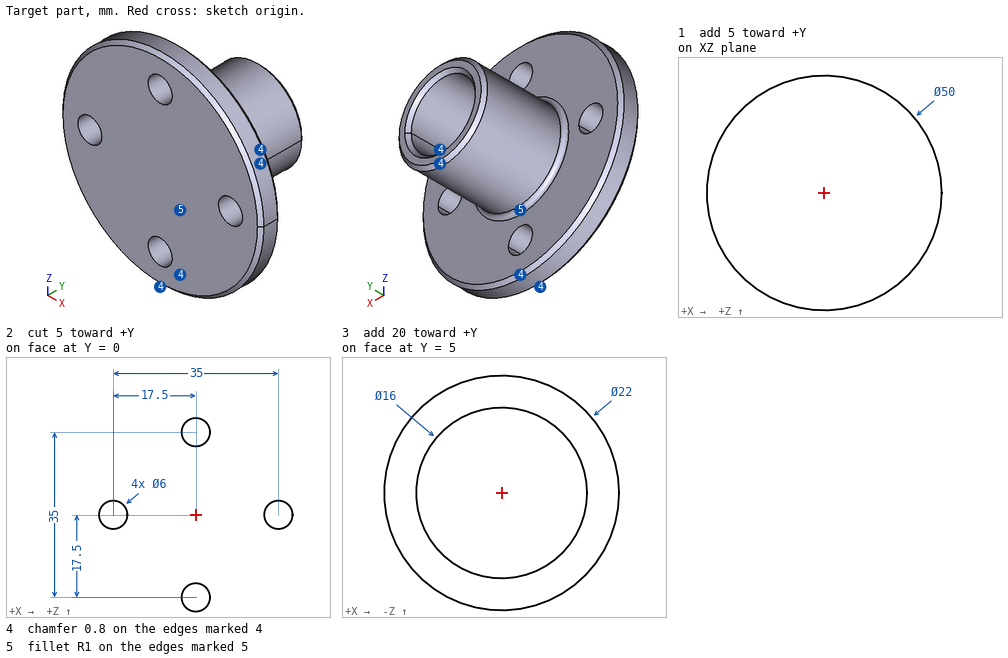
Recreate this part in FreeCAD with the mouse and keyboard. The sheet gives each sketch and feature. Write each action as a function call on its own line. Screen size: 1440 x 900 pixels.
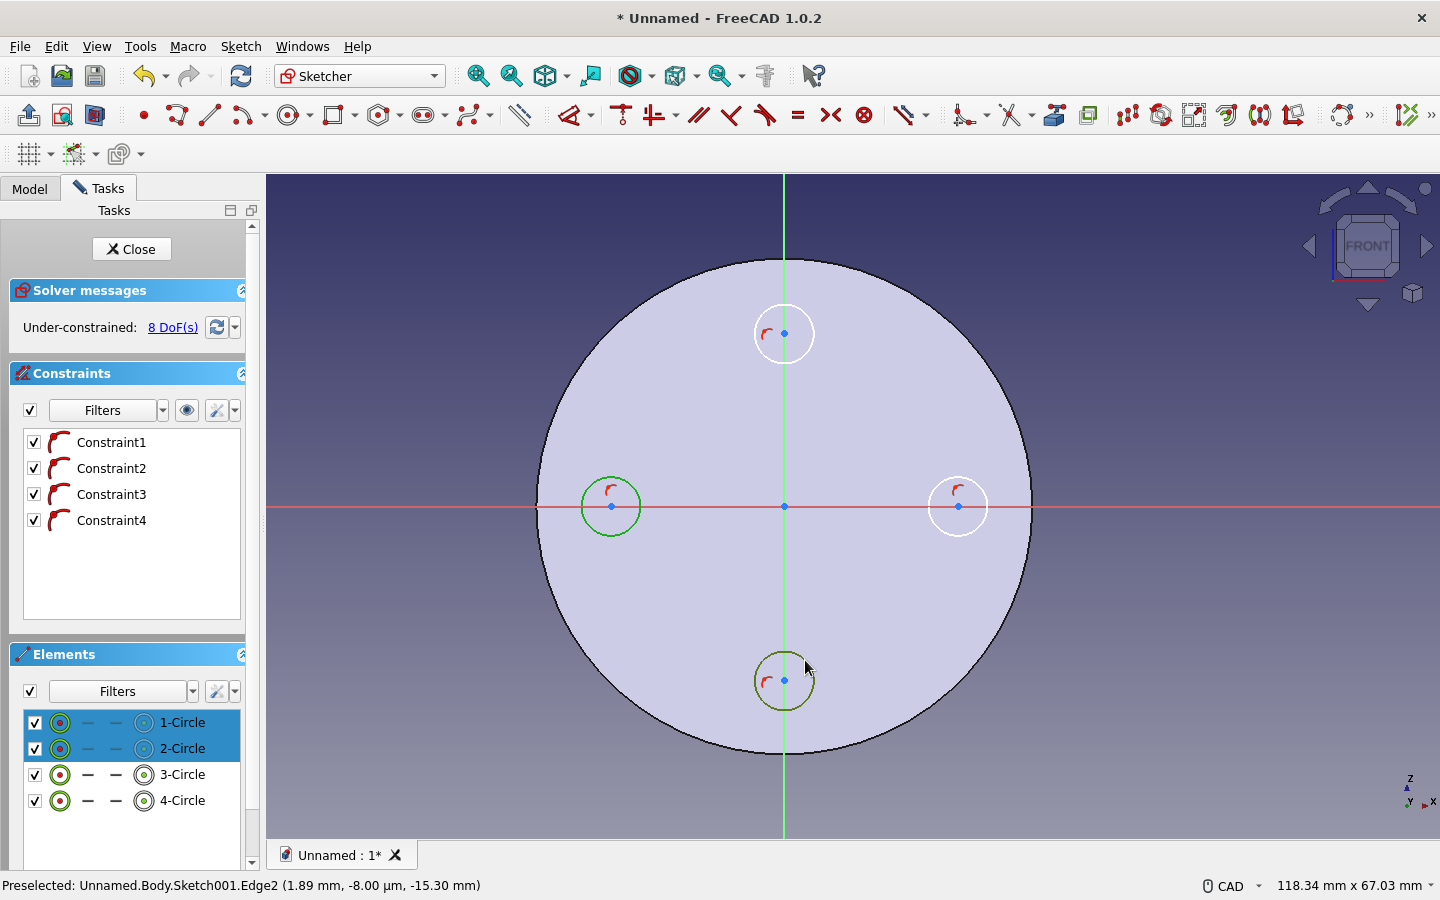
click(979, 486)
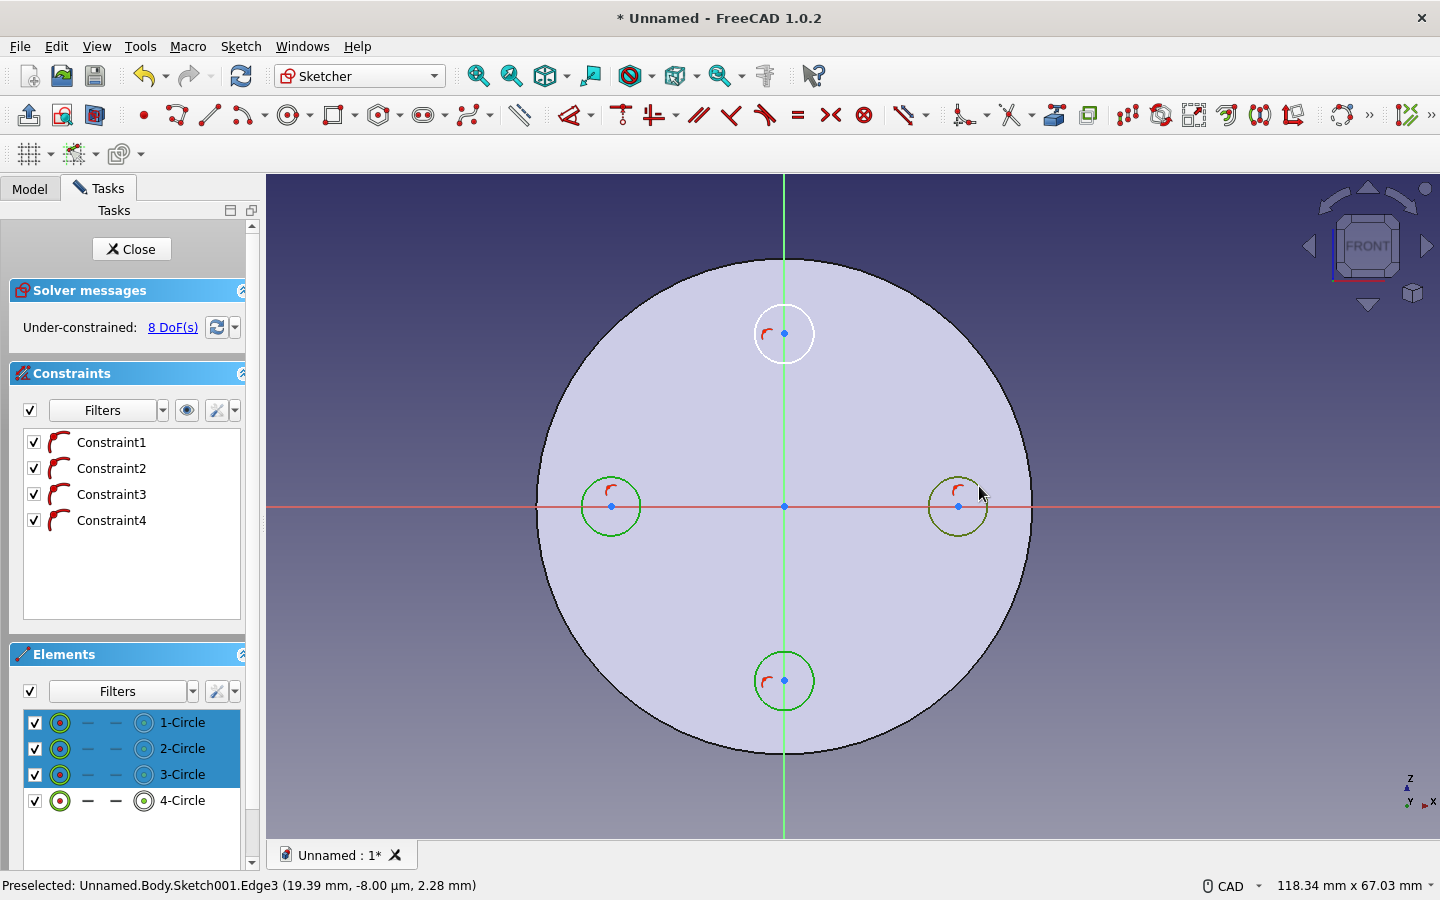
click(805, 313)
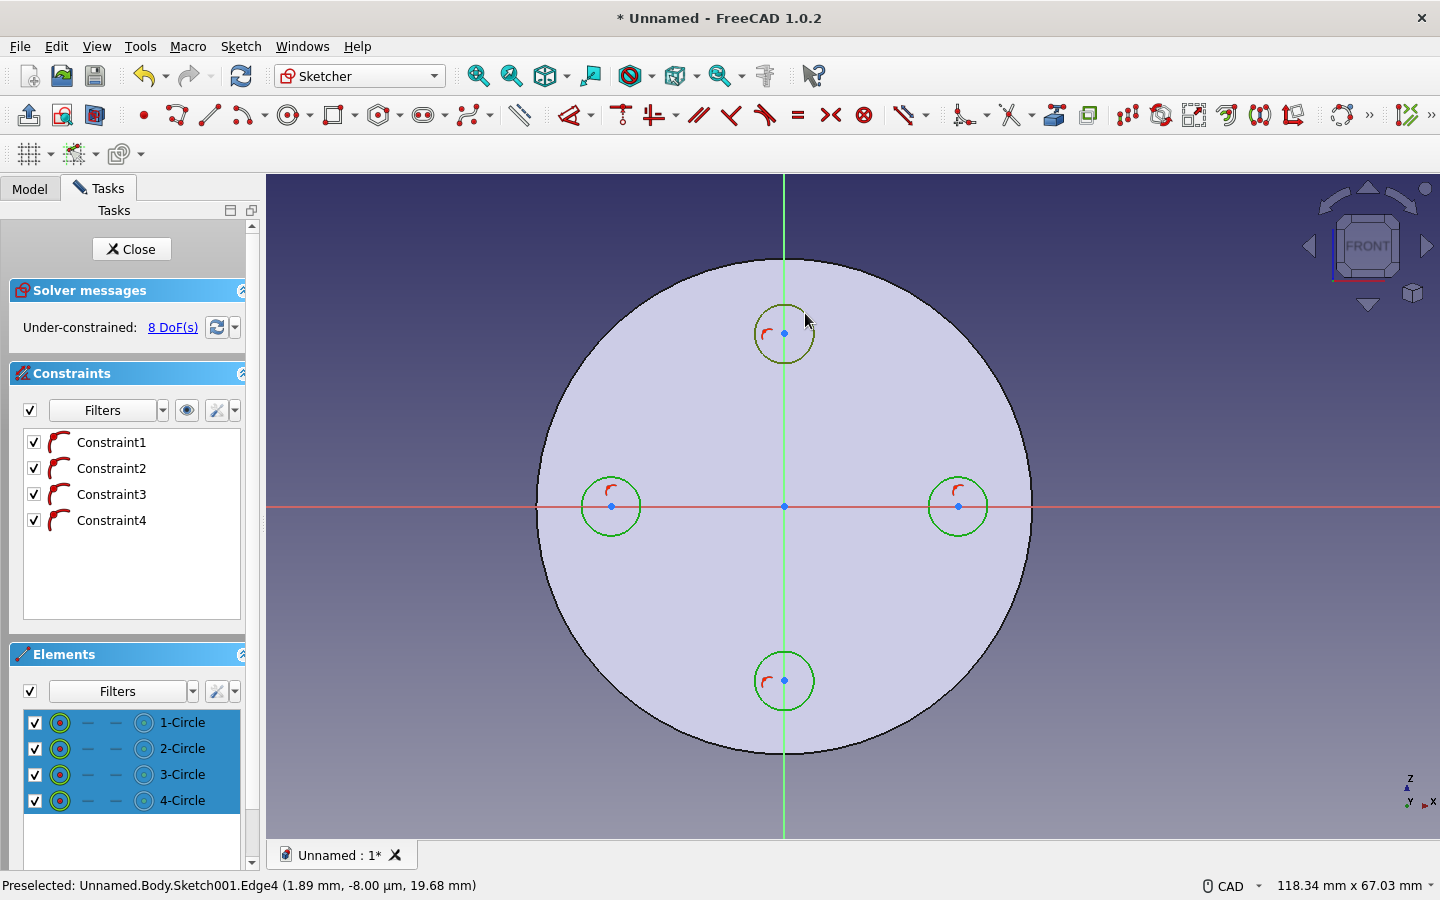
click(798, 116)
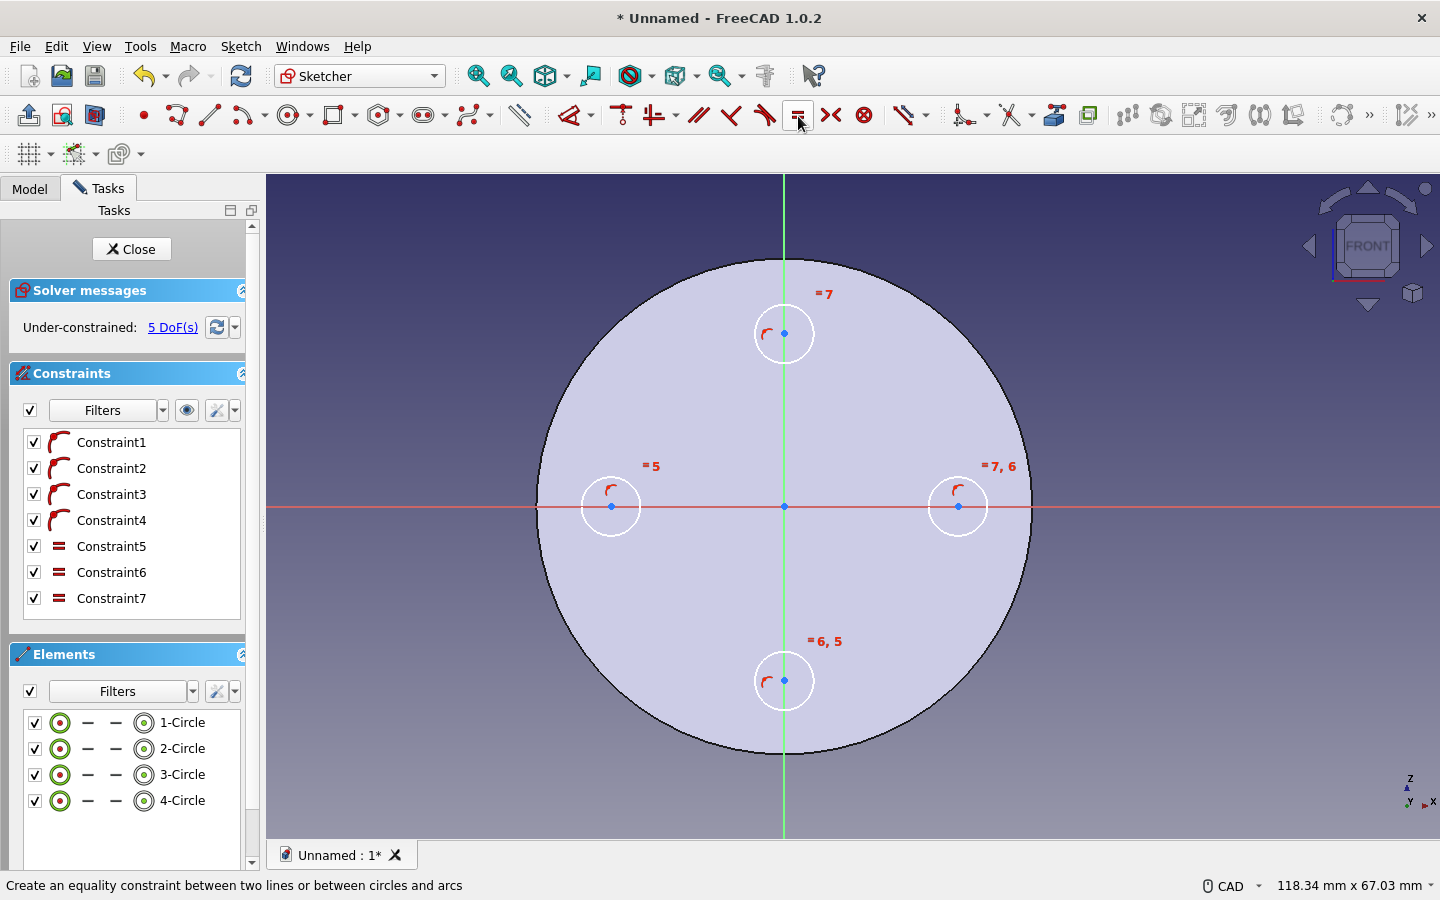
click(568, 116)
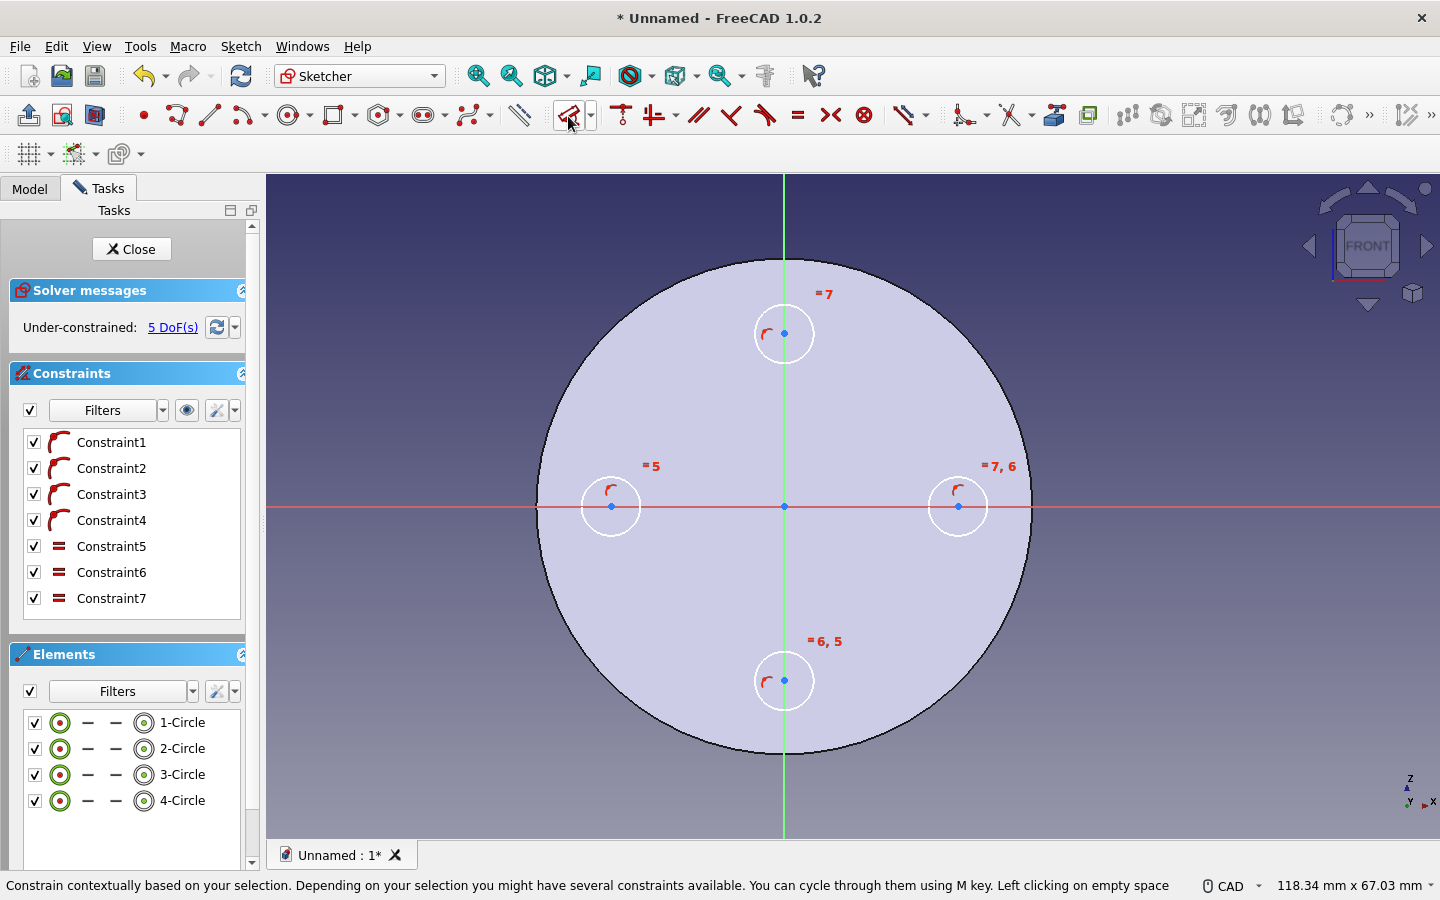
click(632, 486)
click(655, 464)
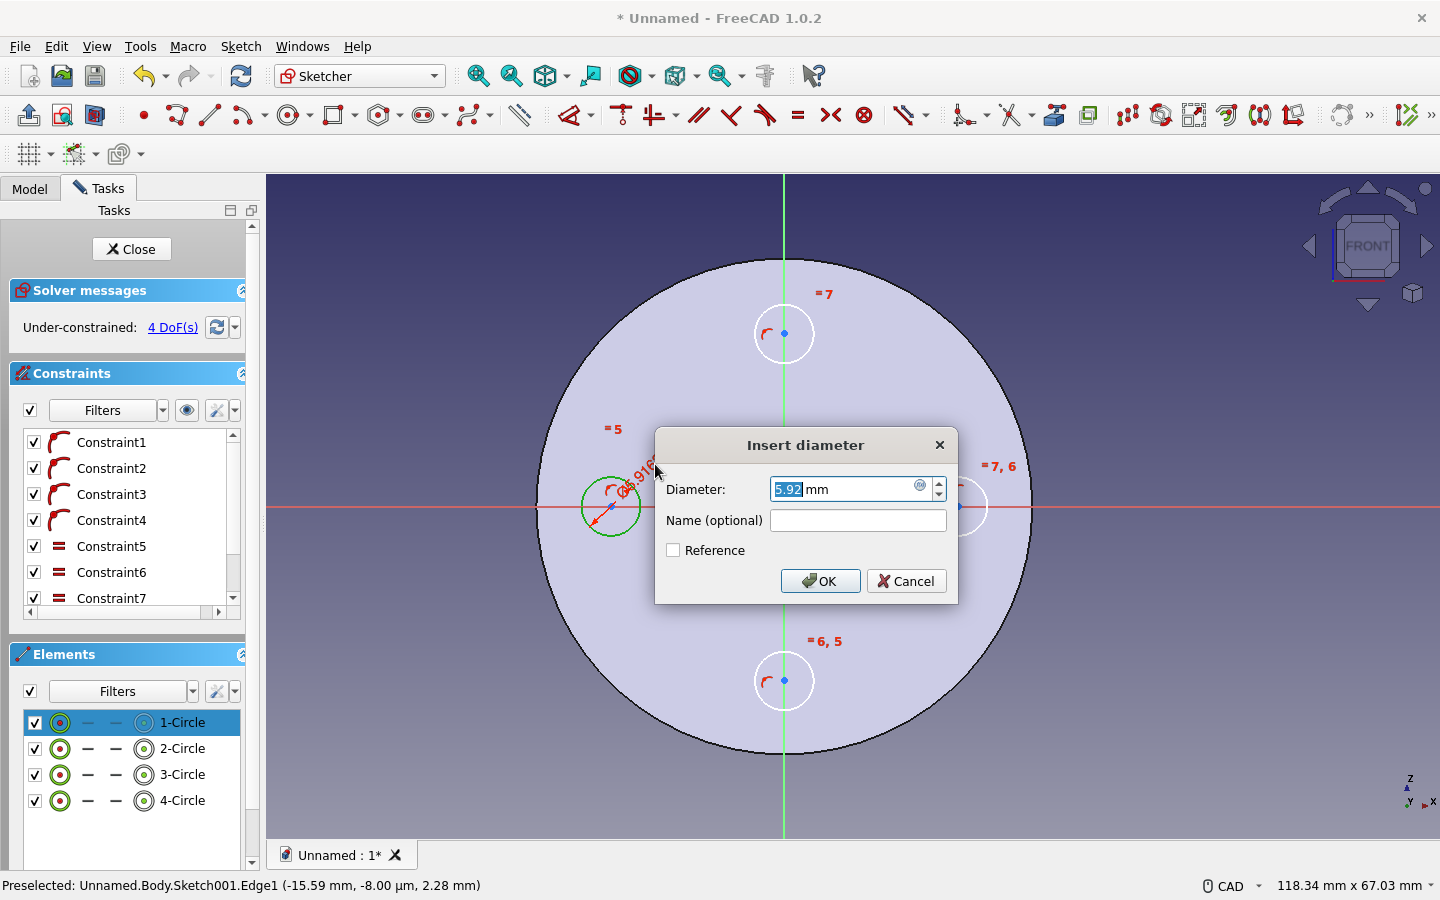
text(6)
key(Return)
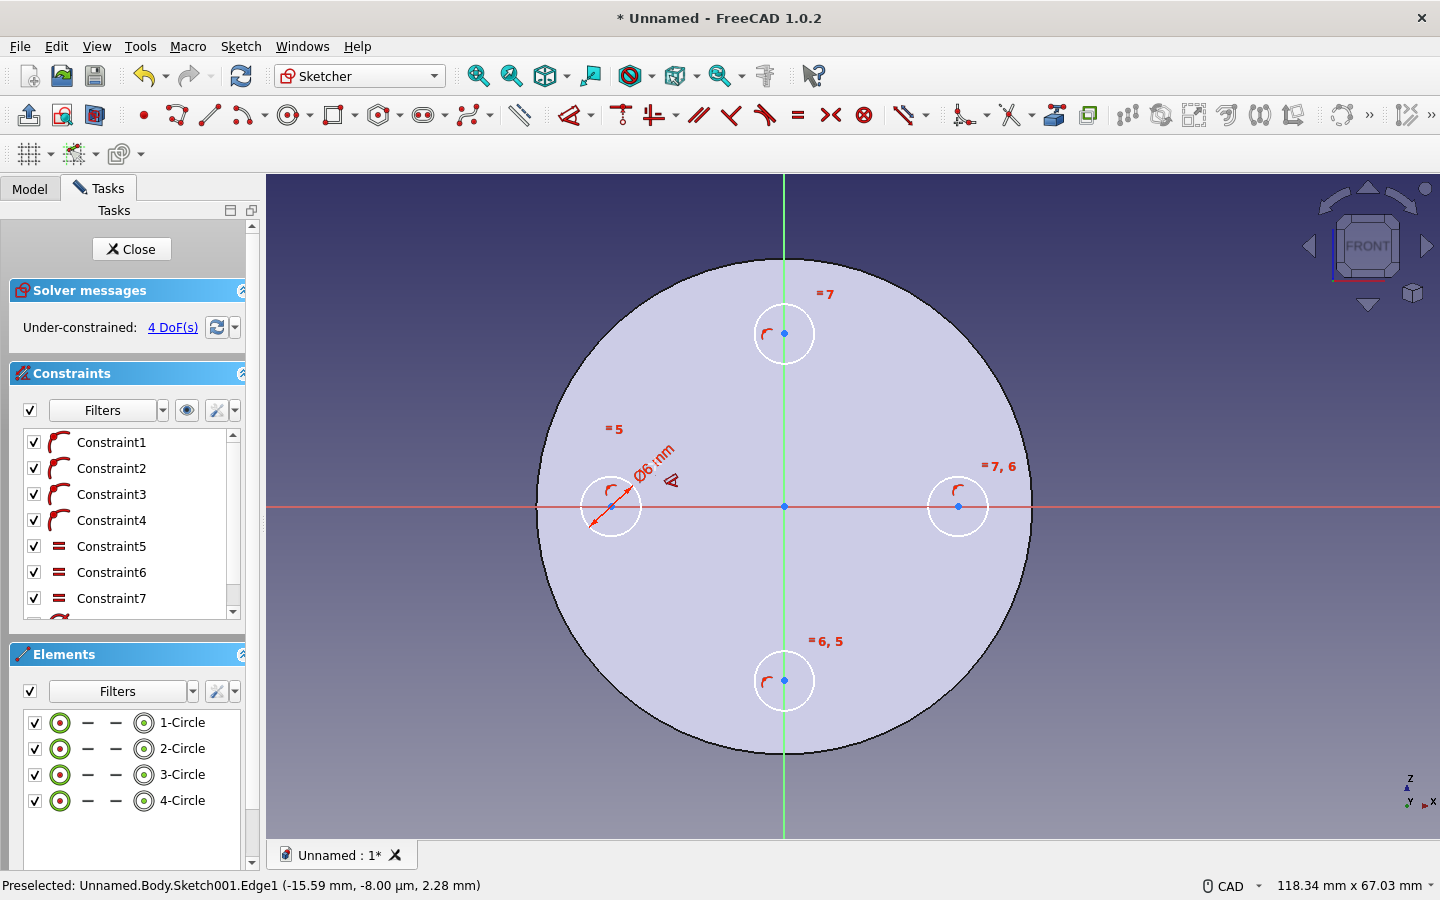
click(611, 506)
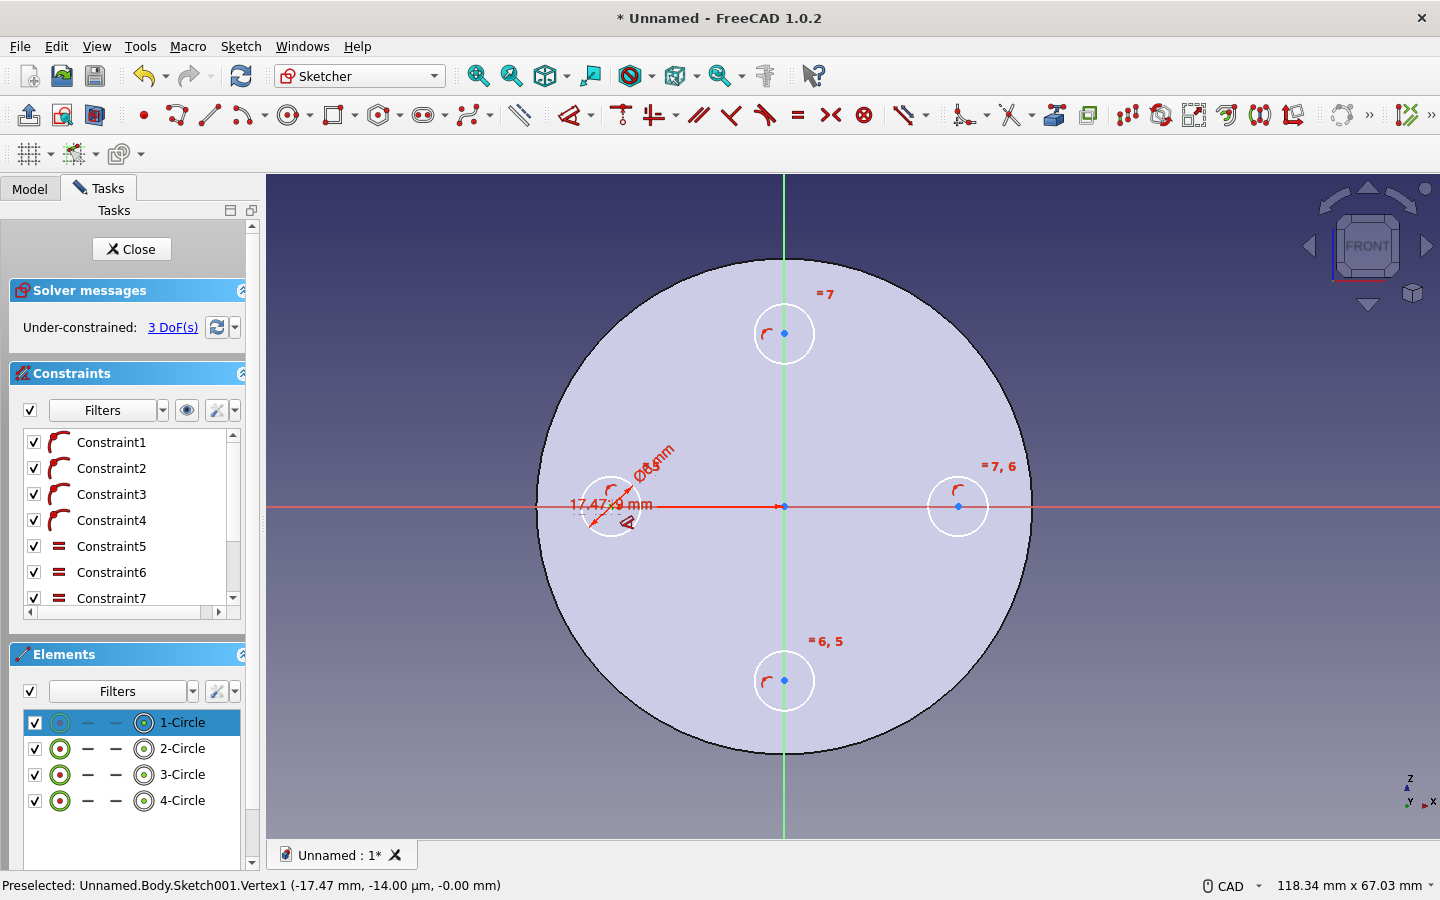
click(958, 506)
click(705, 540)